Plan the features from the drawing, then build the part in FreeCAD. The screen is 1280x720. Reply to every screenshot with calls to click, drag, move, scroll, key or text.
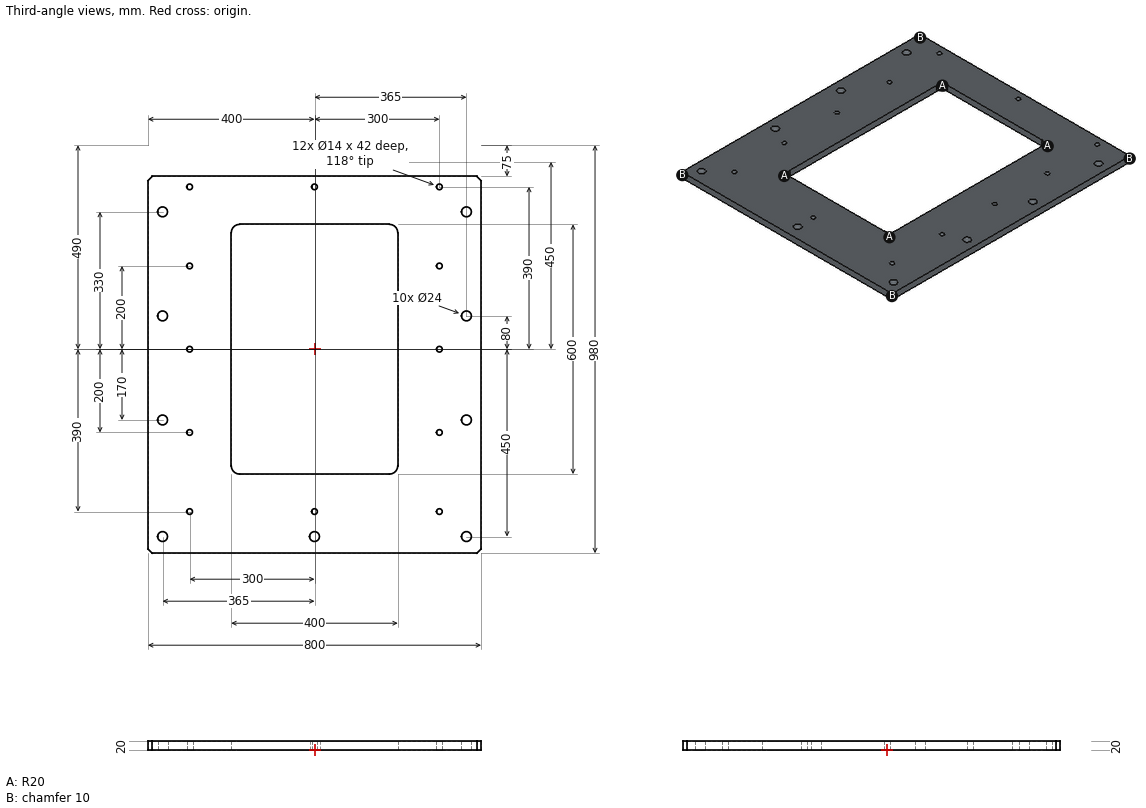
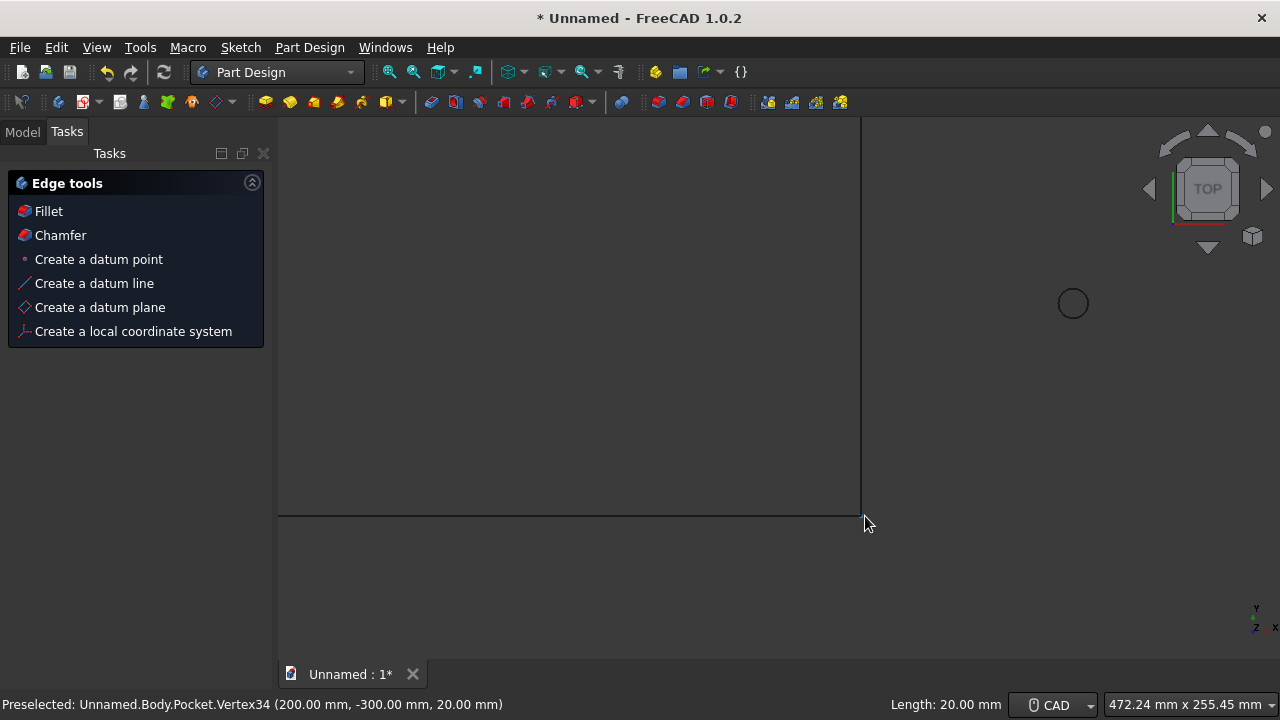
click(390, 72)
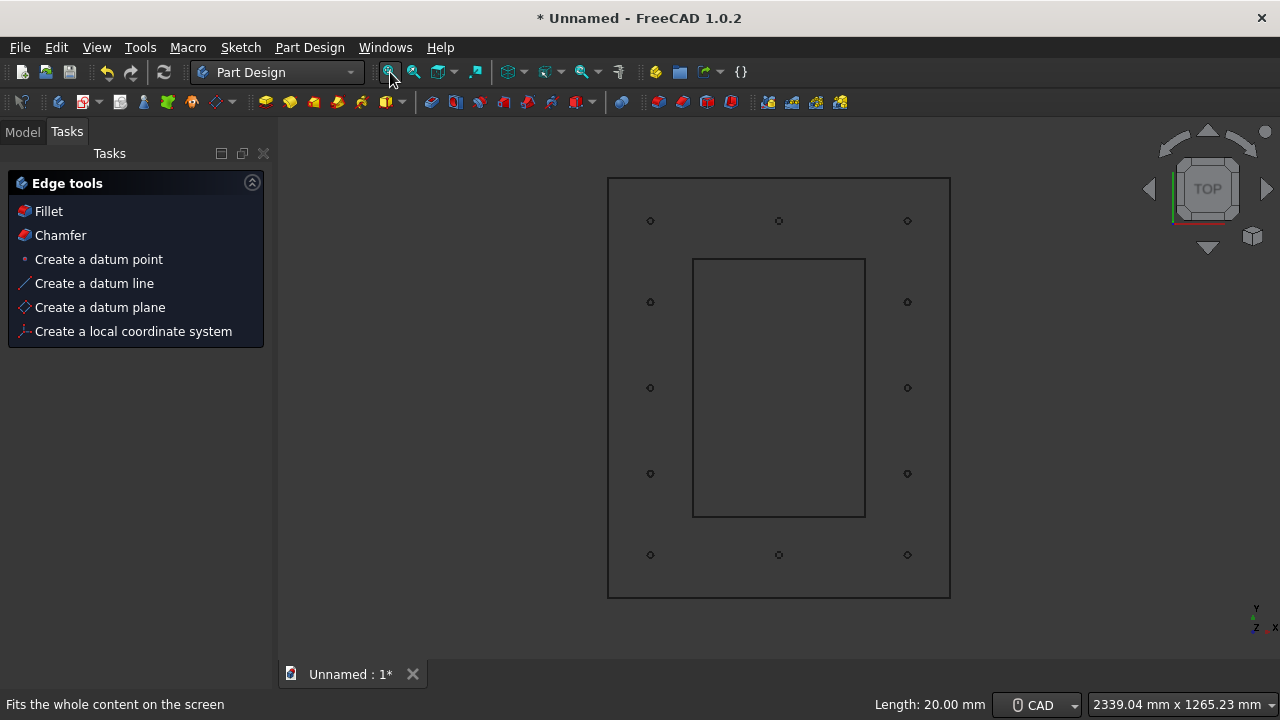
key(1)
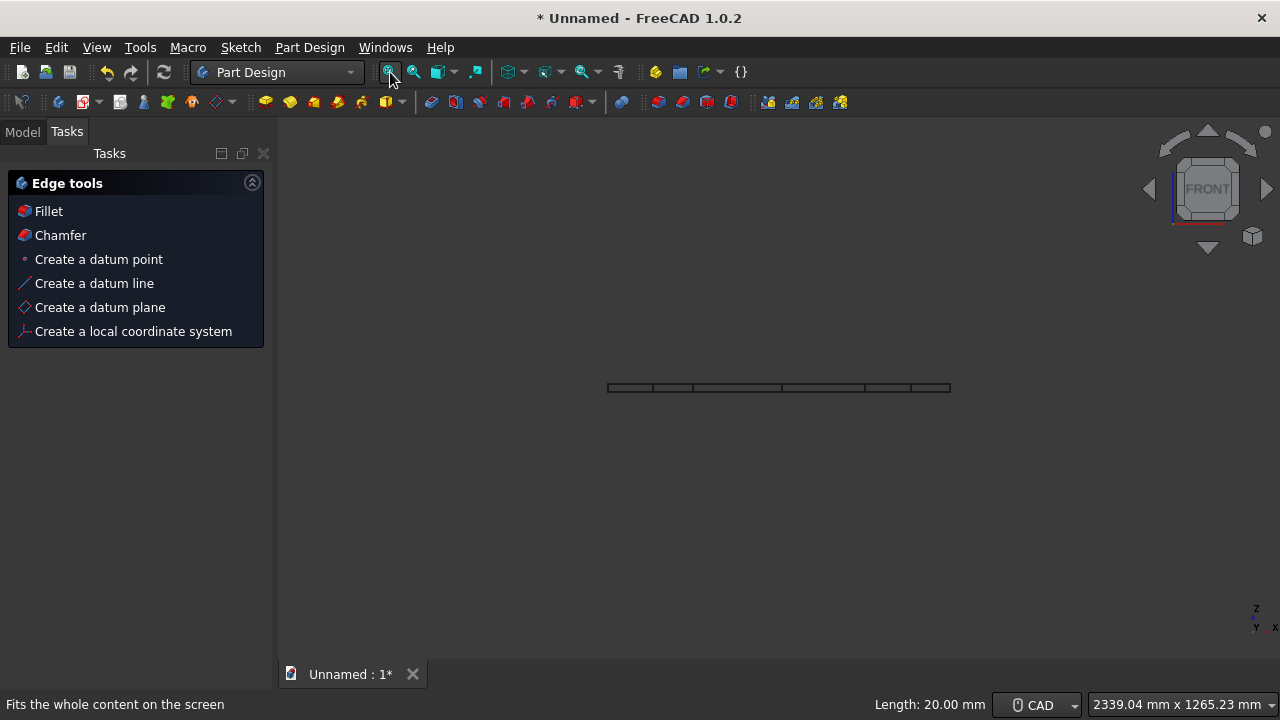
click(390, 72)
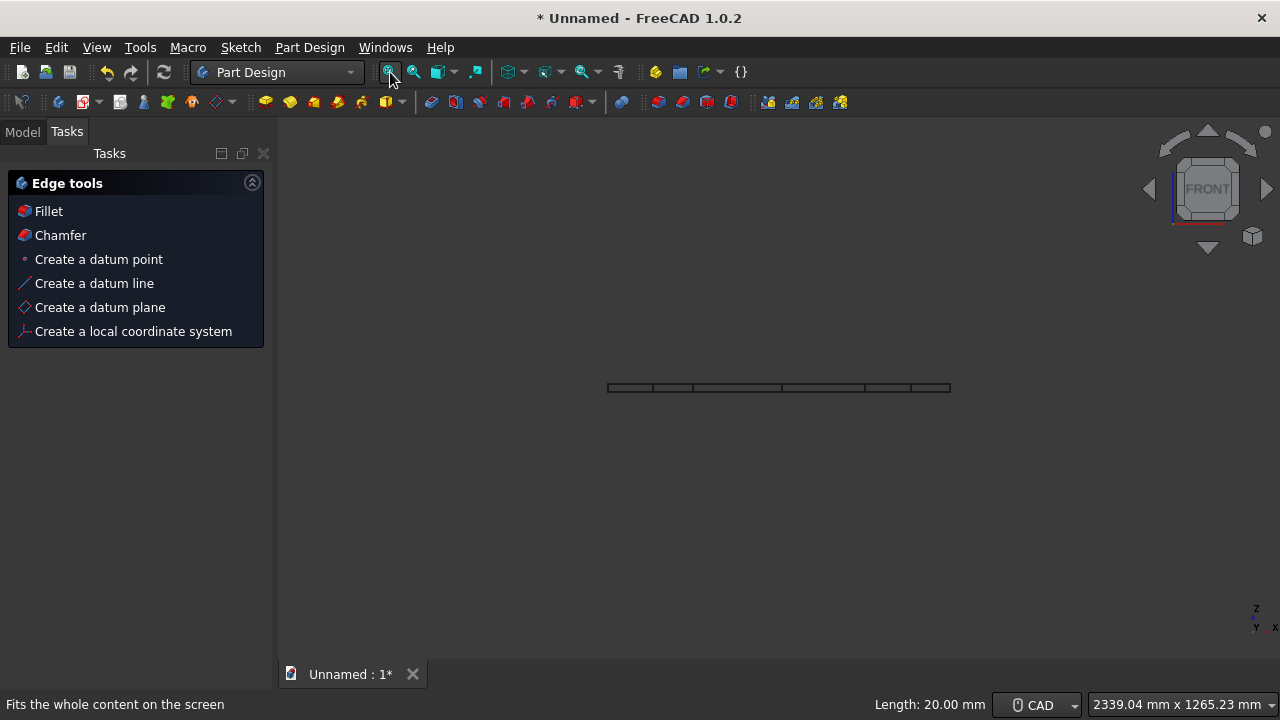
scroll(865, 387, up, 8)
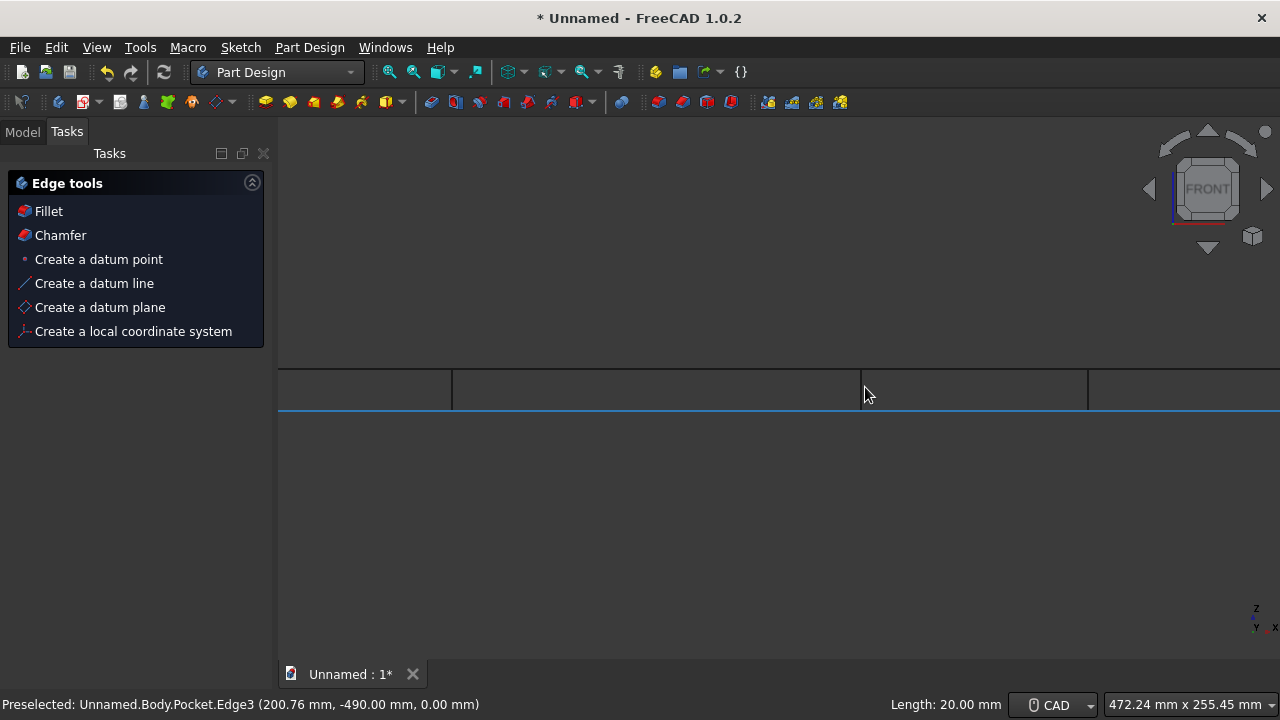
click(861, 389, ctrl)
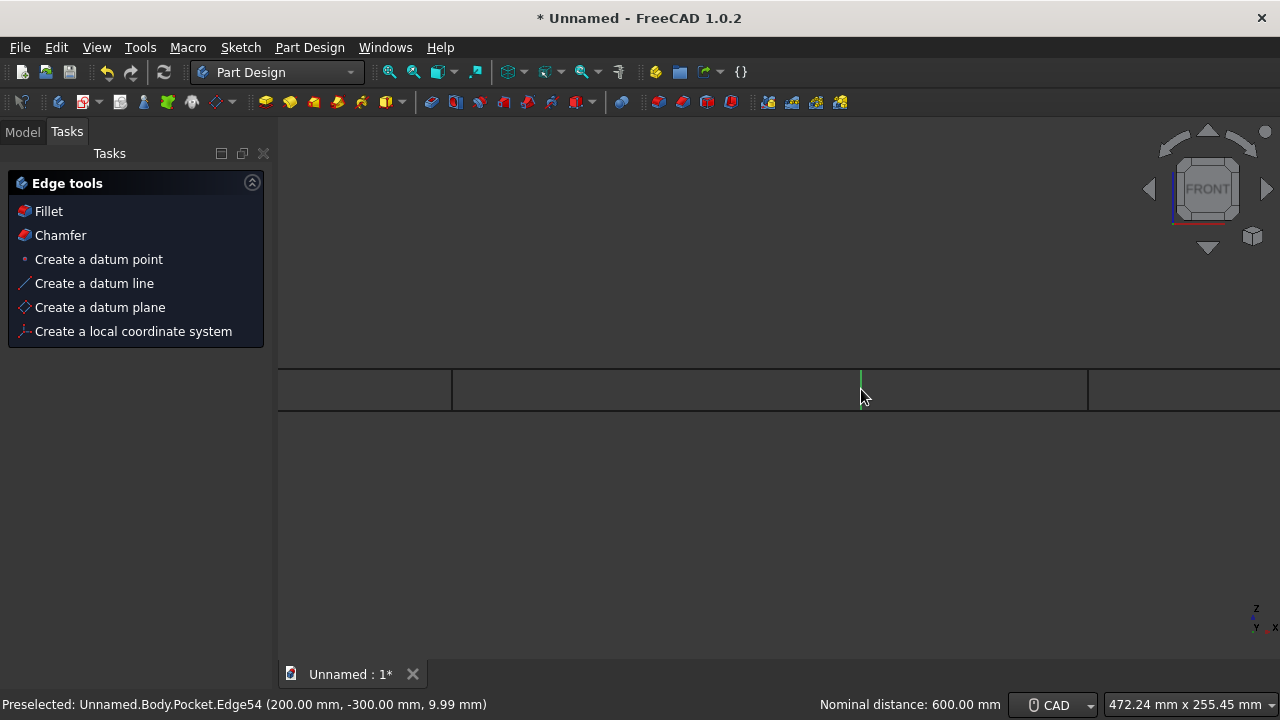
click(390, 72)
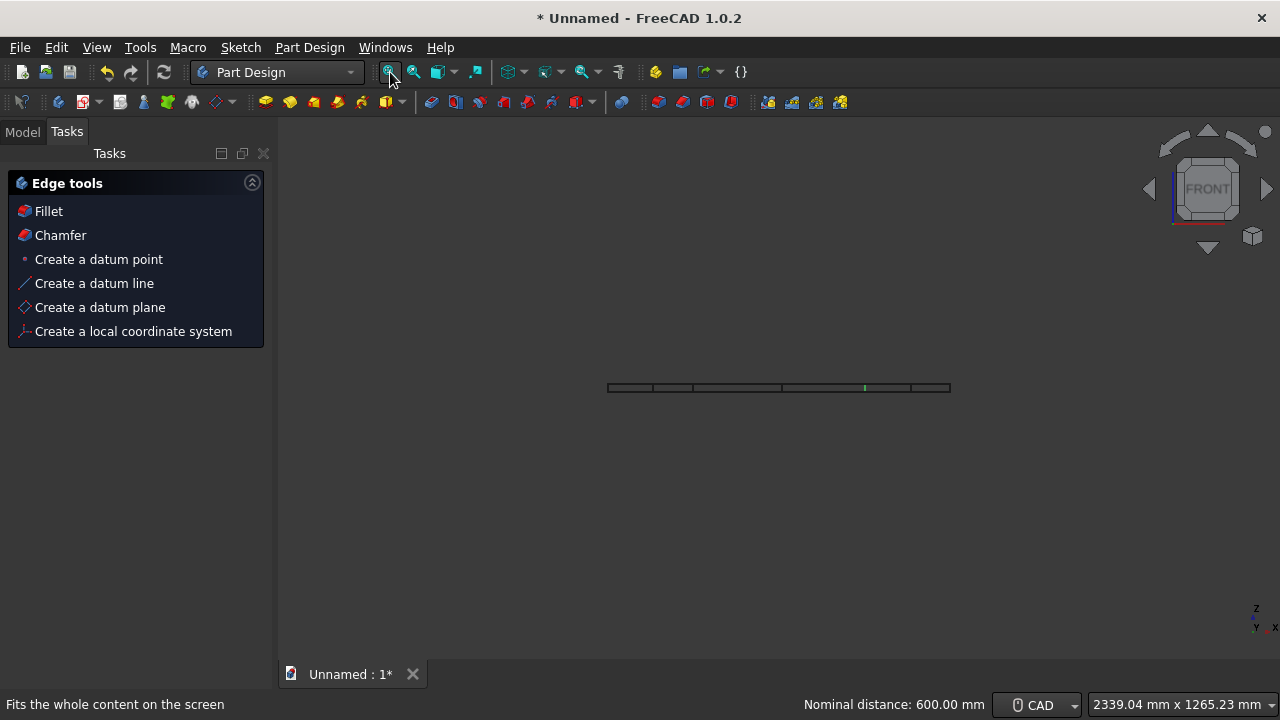
key(3)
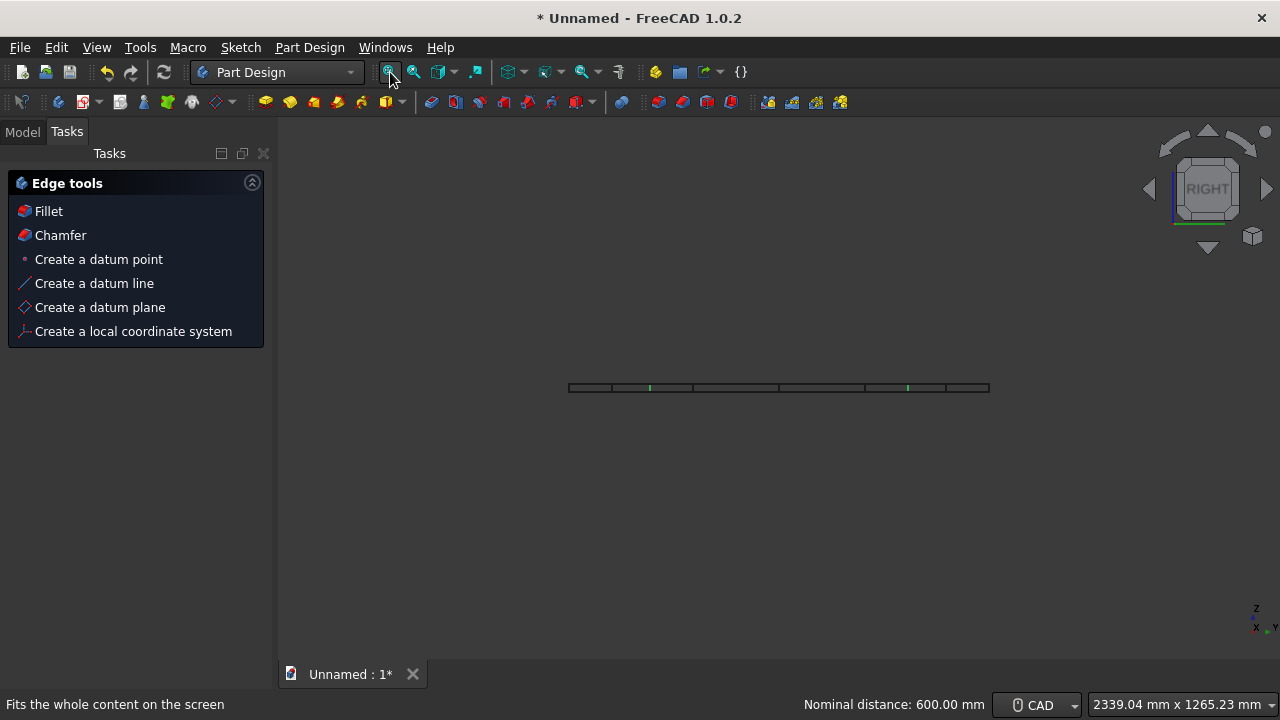
click(390, 72)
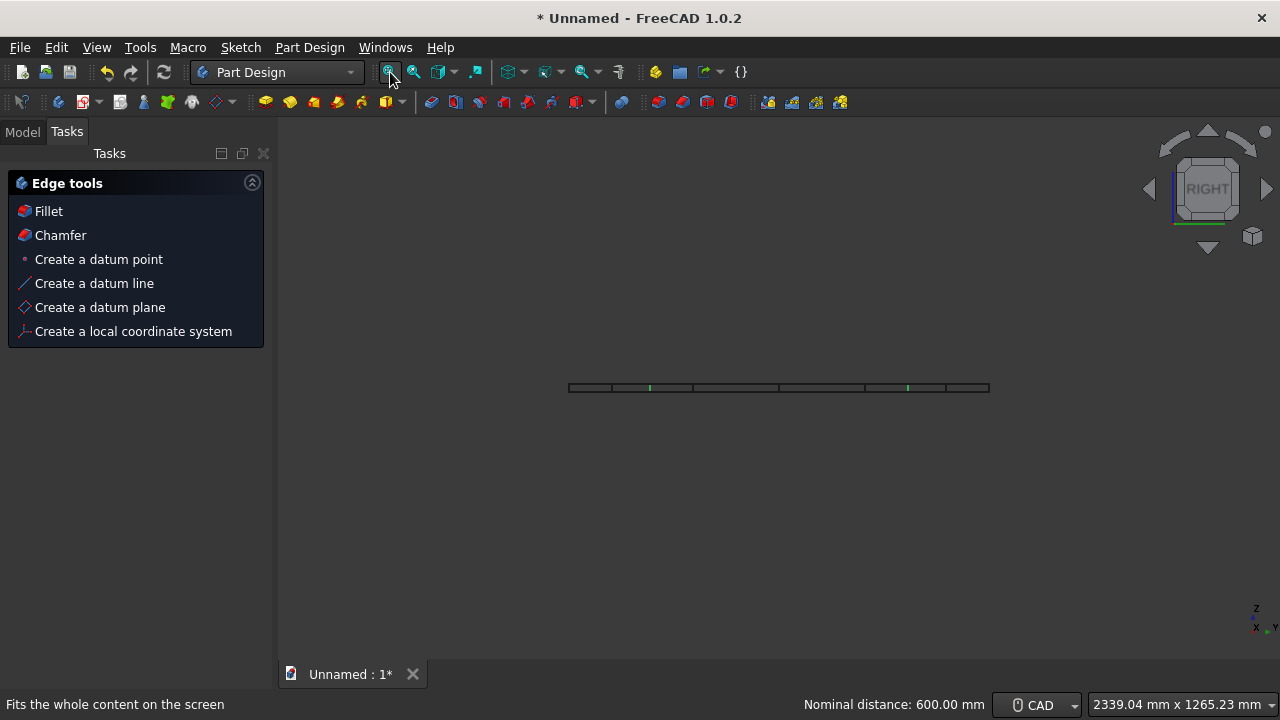
scroll(650, 387, up, 8)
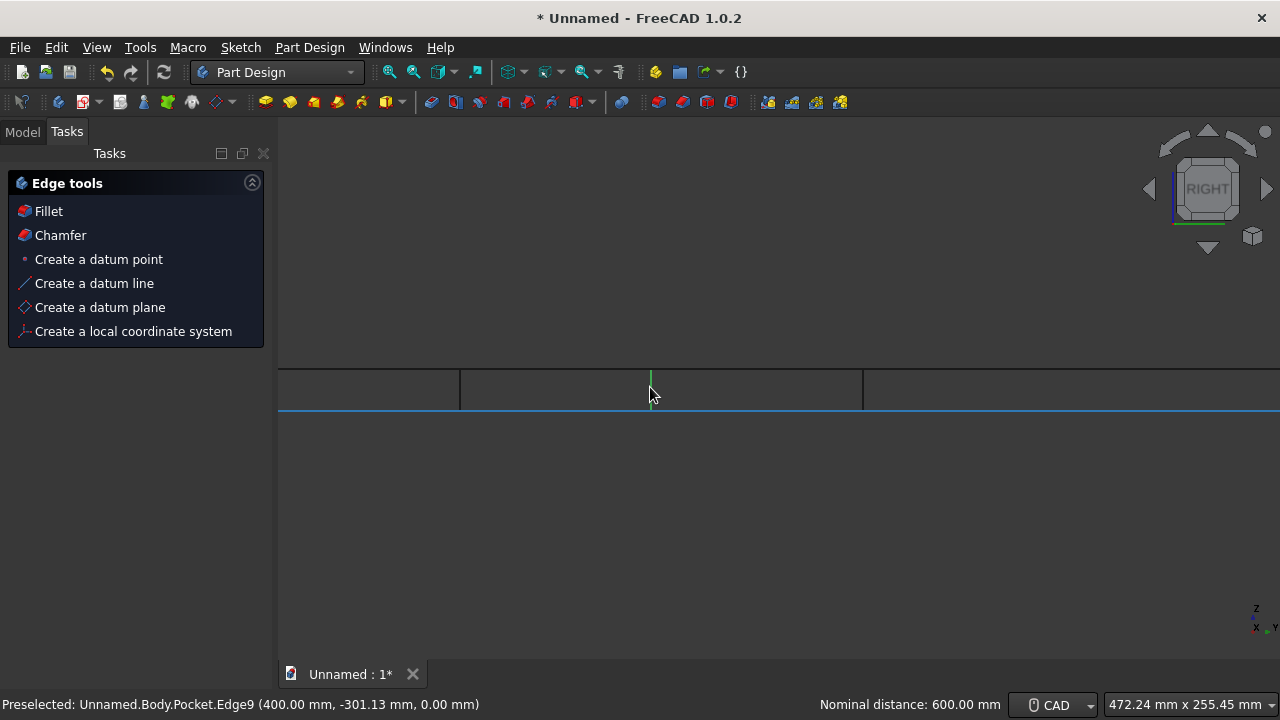
click(390, 72)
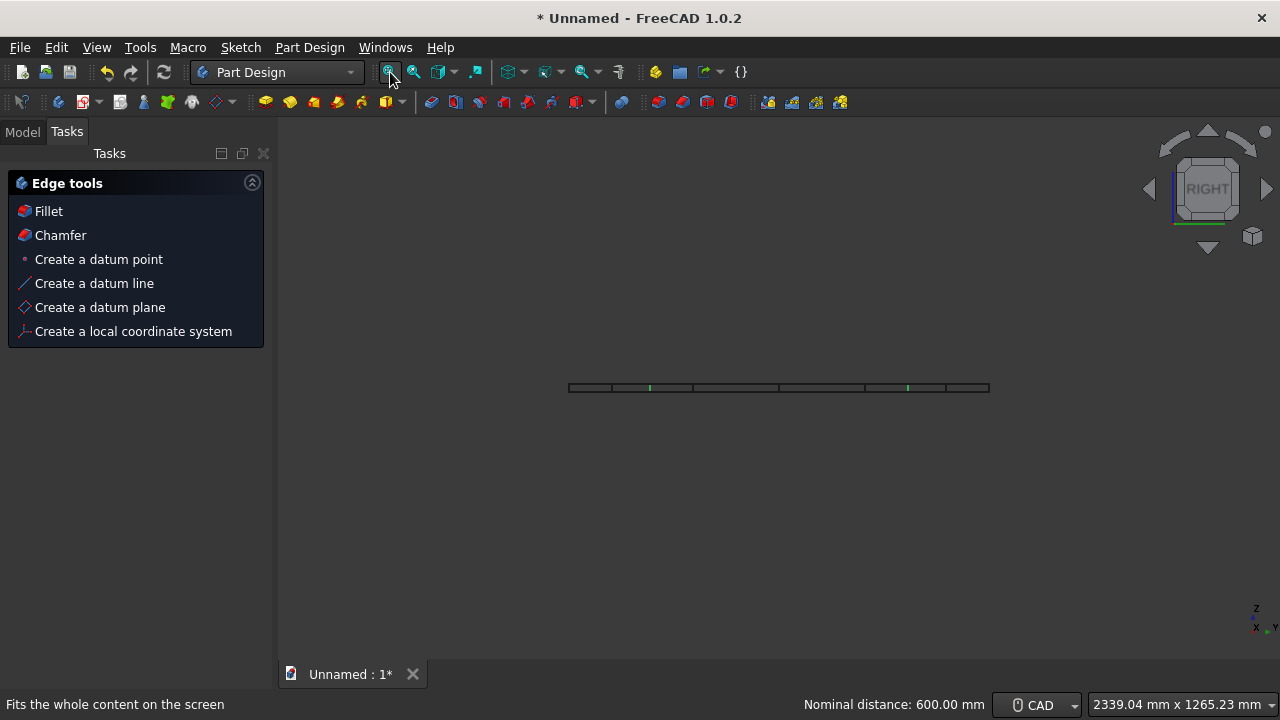
key(5)